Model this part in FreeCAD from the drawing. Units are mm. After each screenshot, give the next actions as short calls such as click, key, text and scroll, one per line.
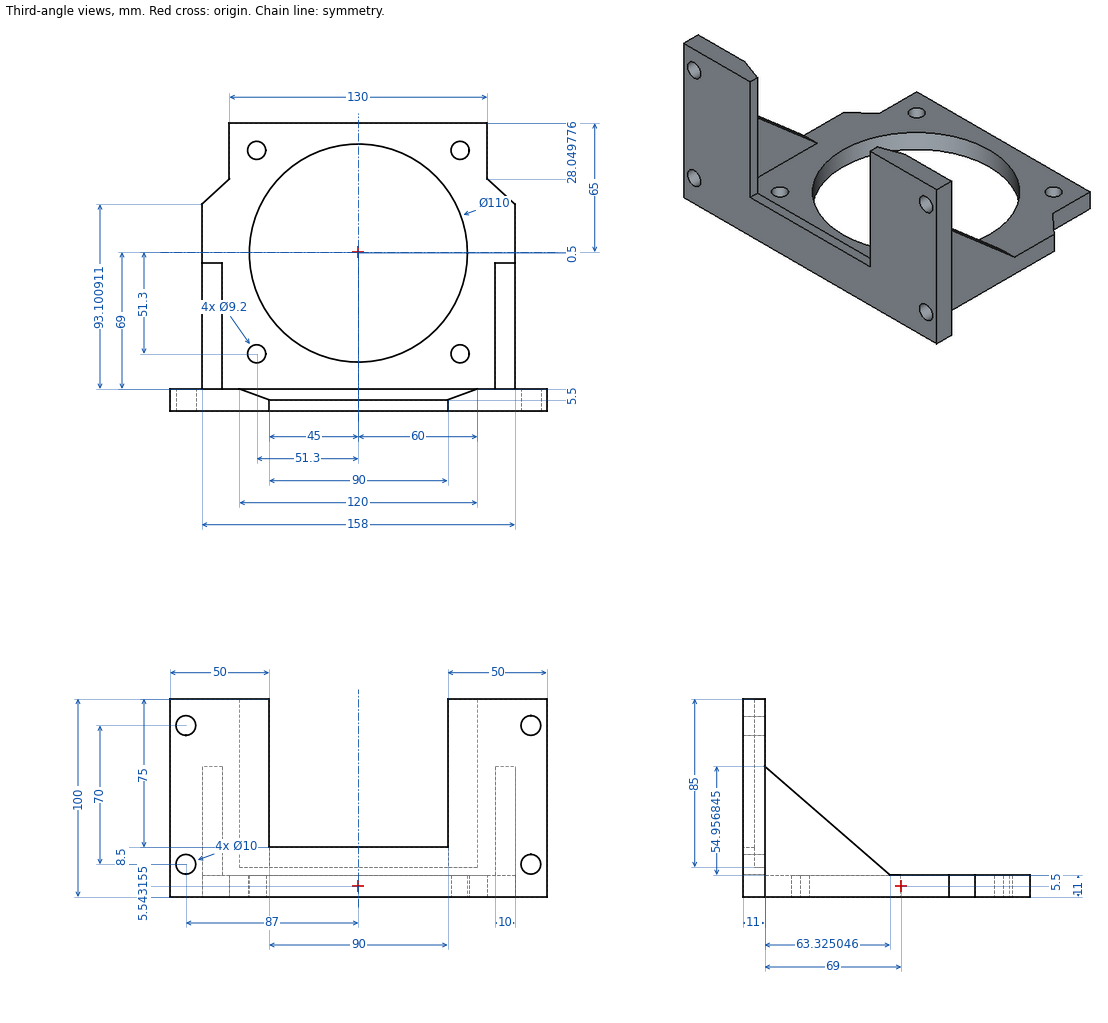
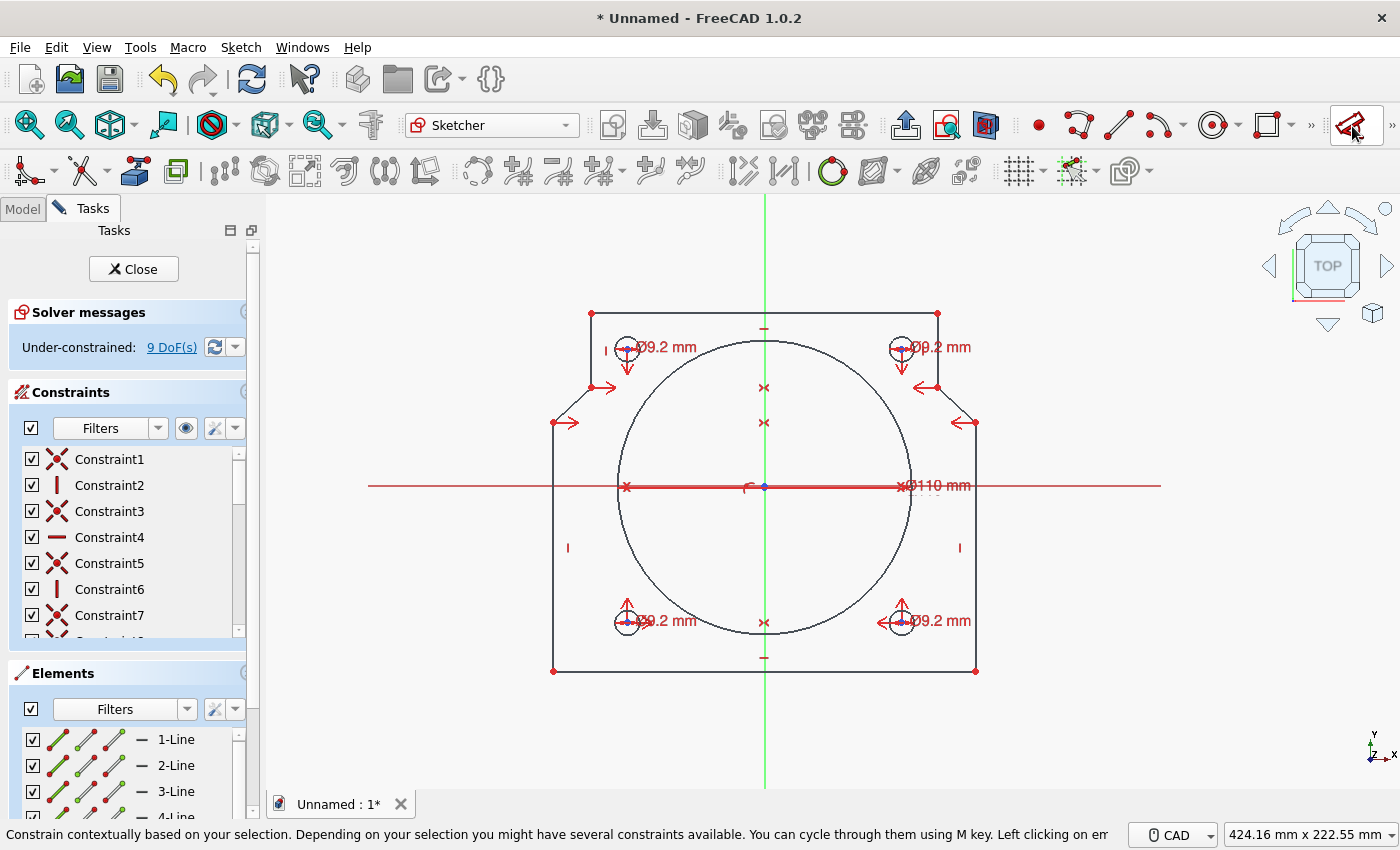
click(680, 672)
click(667, 706)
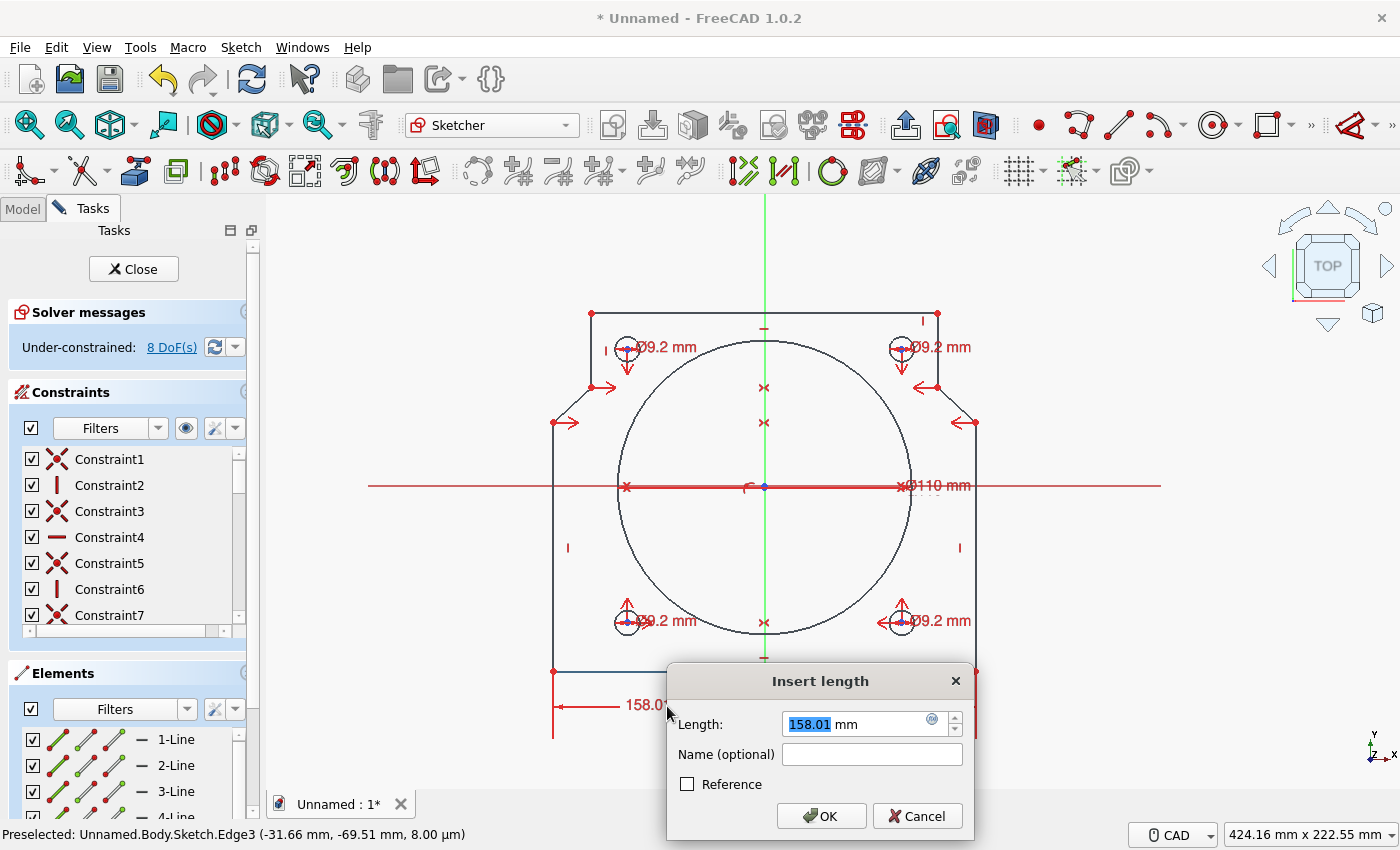
text(158)
key(Return)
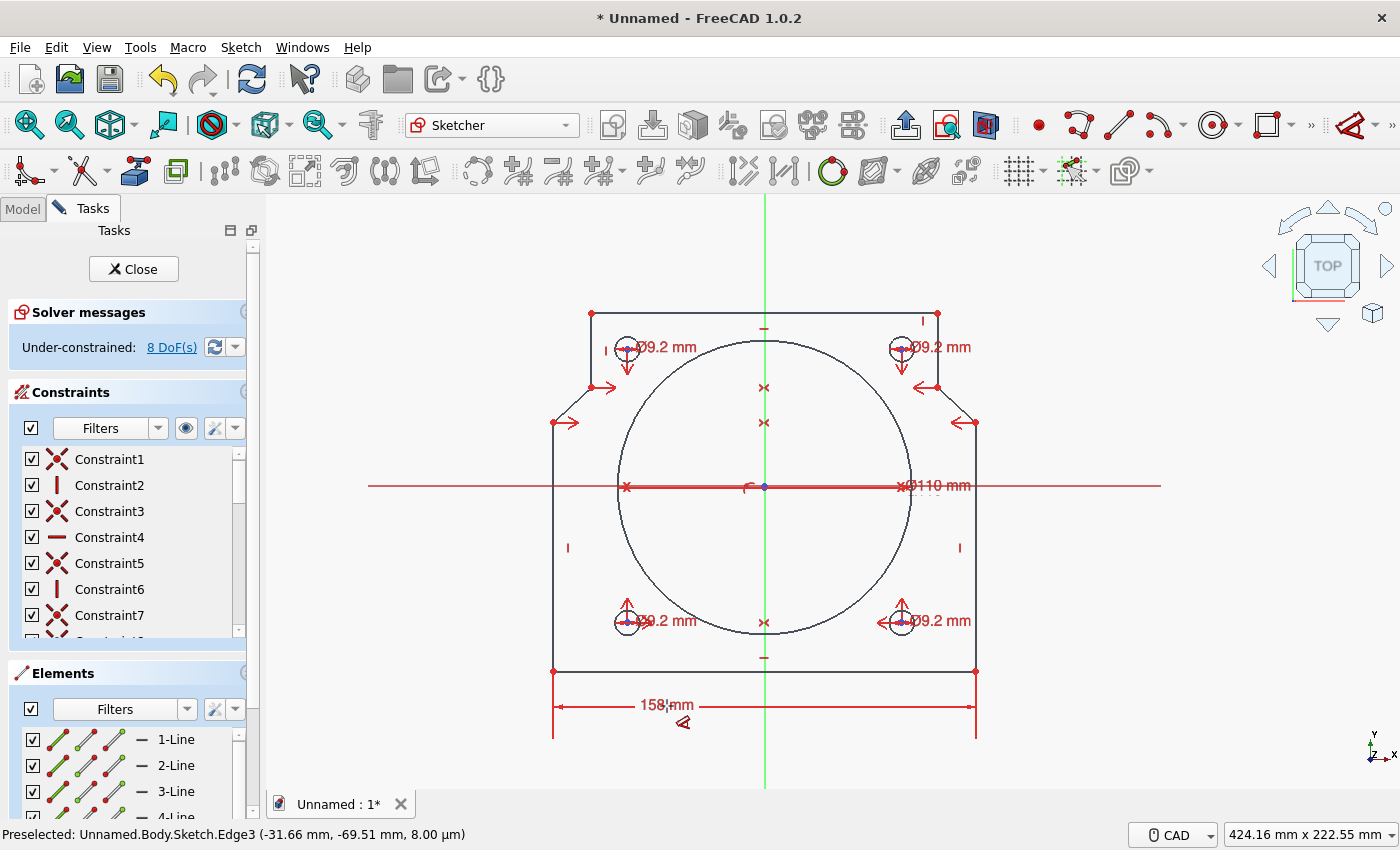
click(834, 313)
click(685, 279)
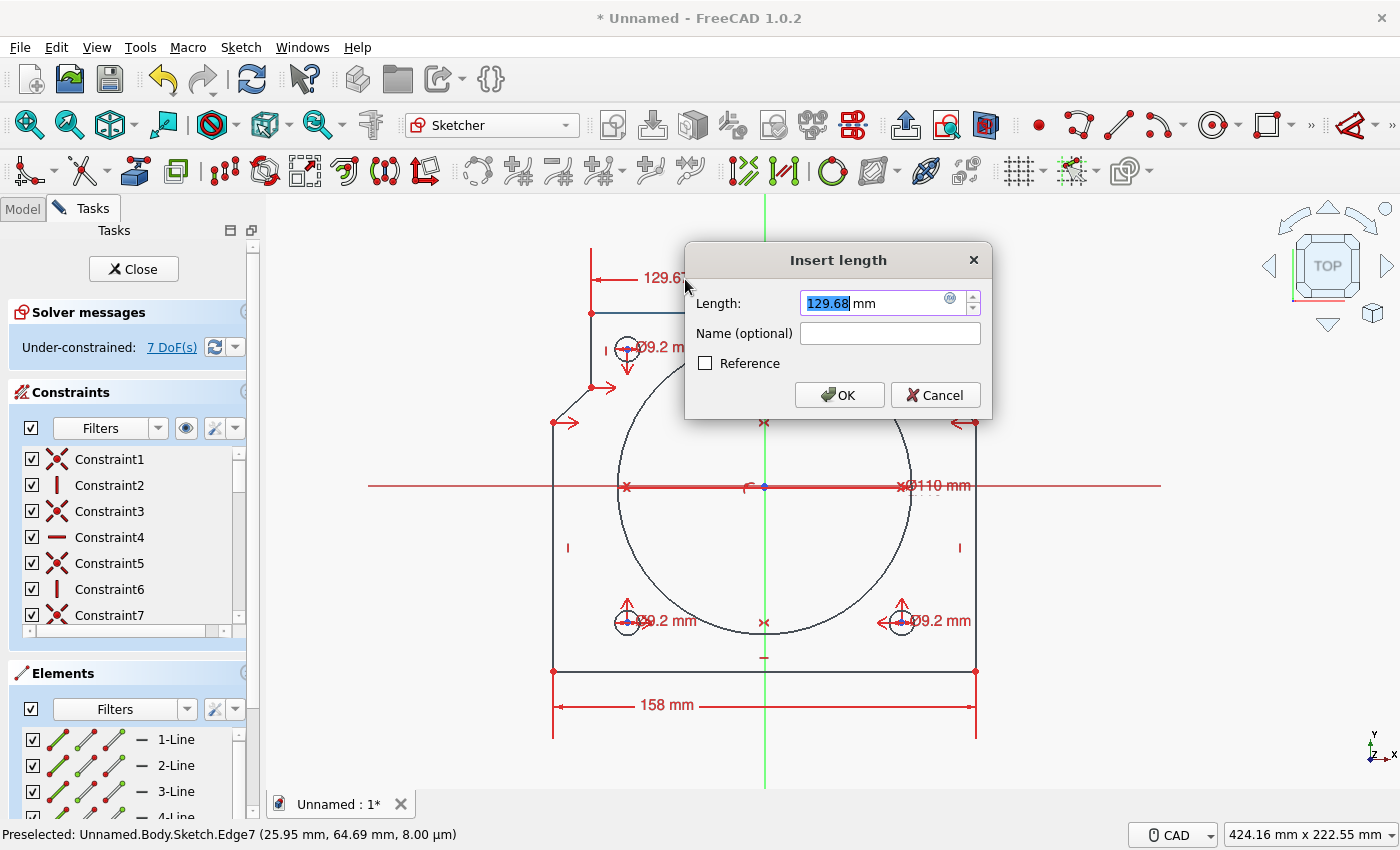
text(130)
key(Return)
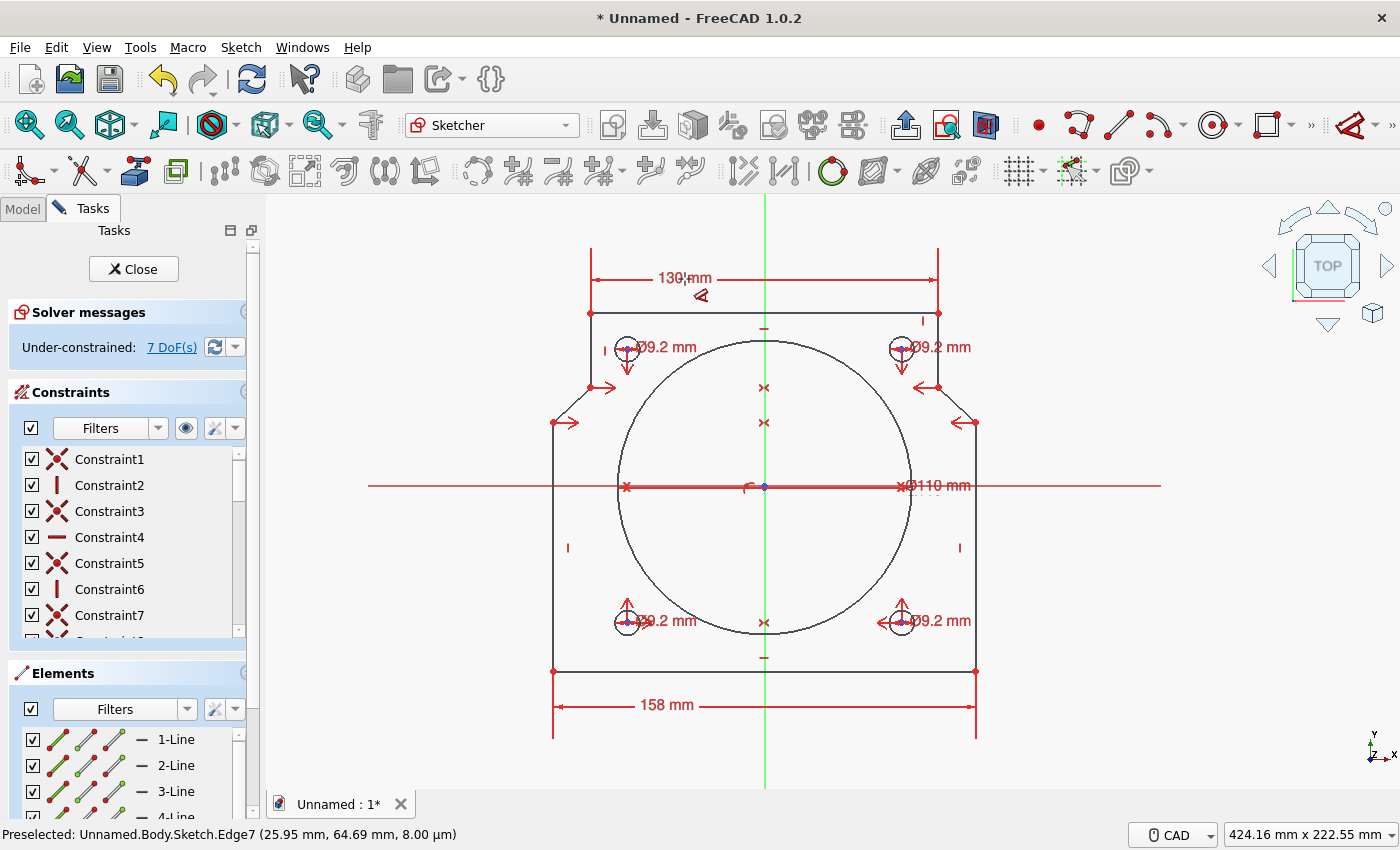
click(553, 672)
click(519, 579)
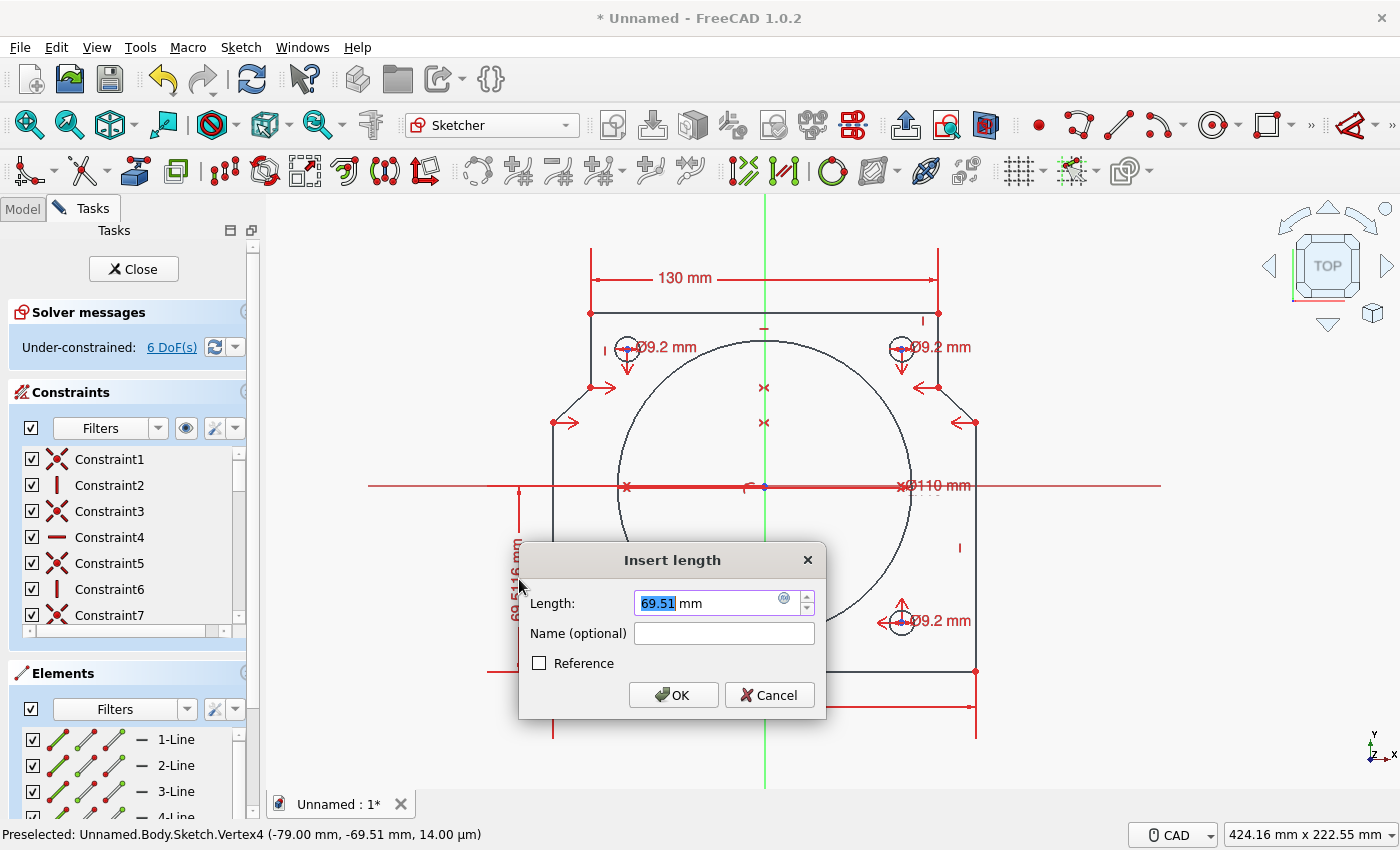
text(69)
key(Return)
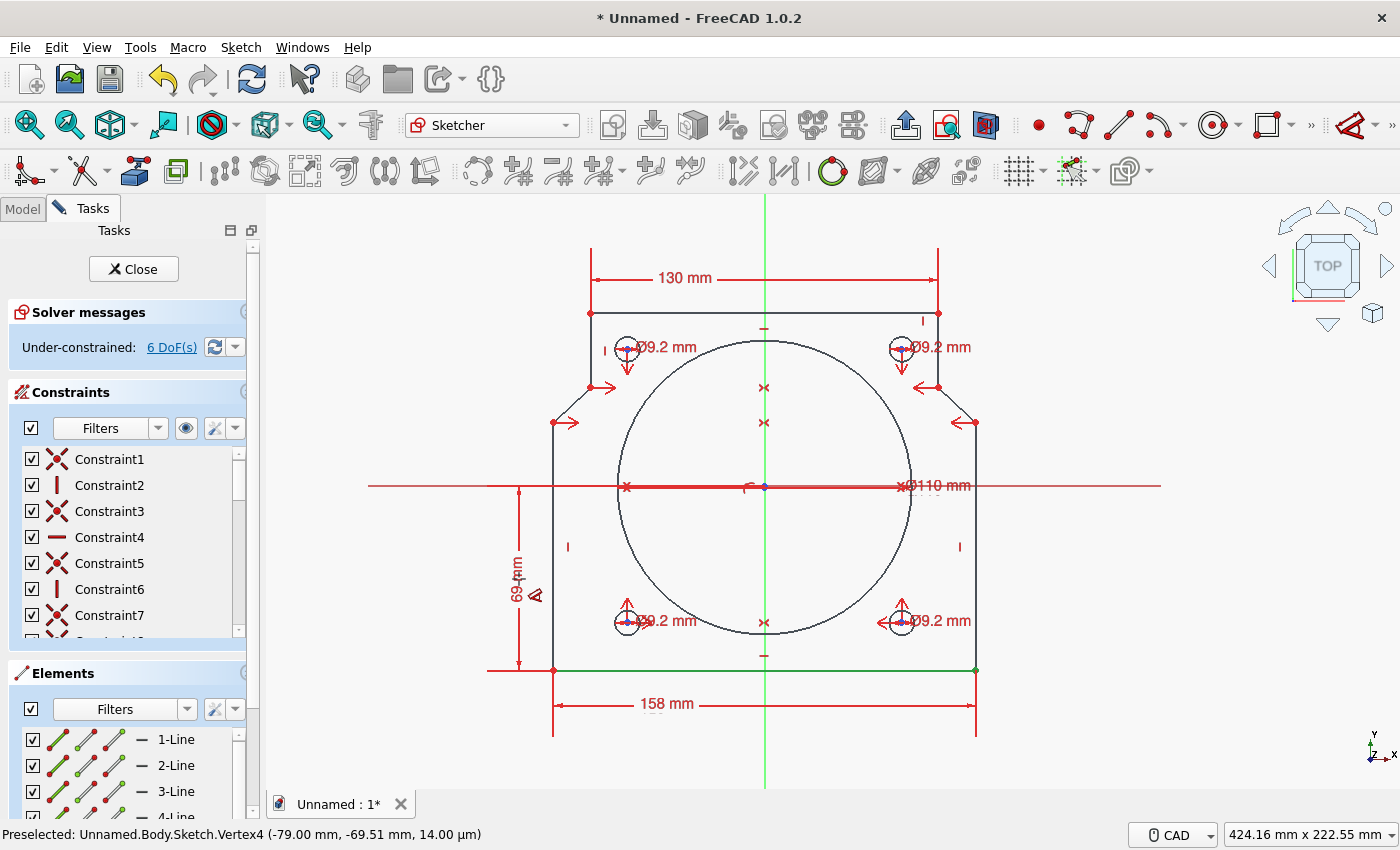
click(938, 313)
click(972, 400)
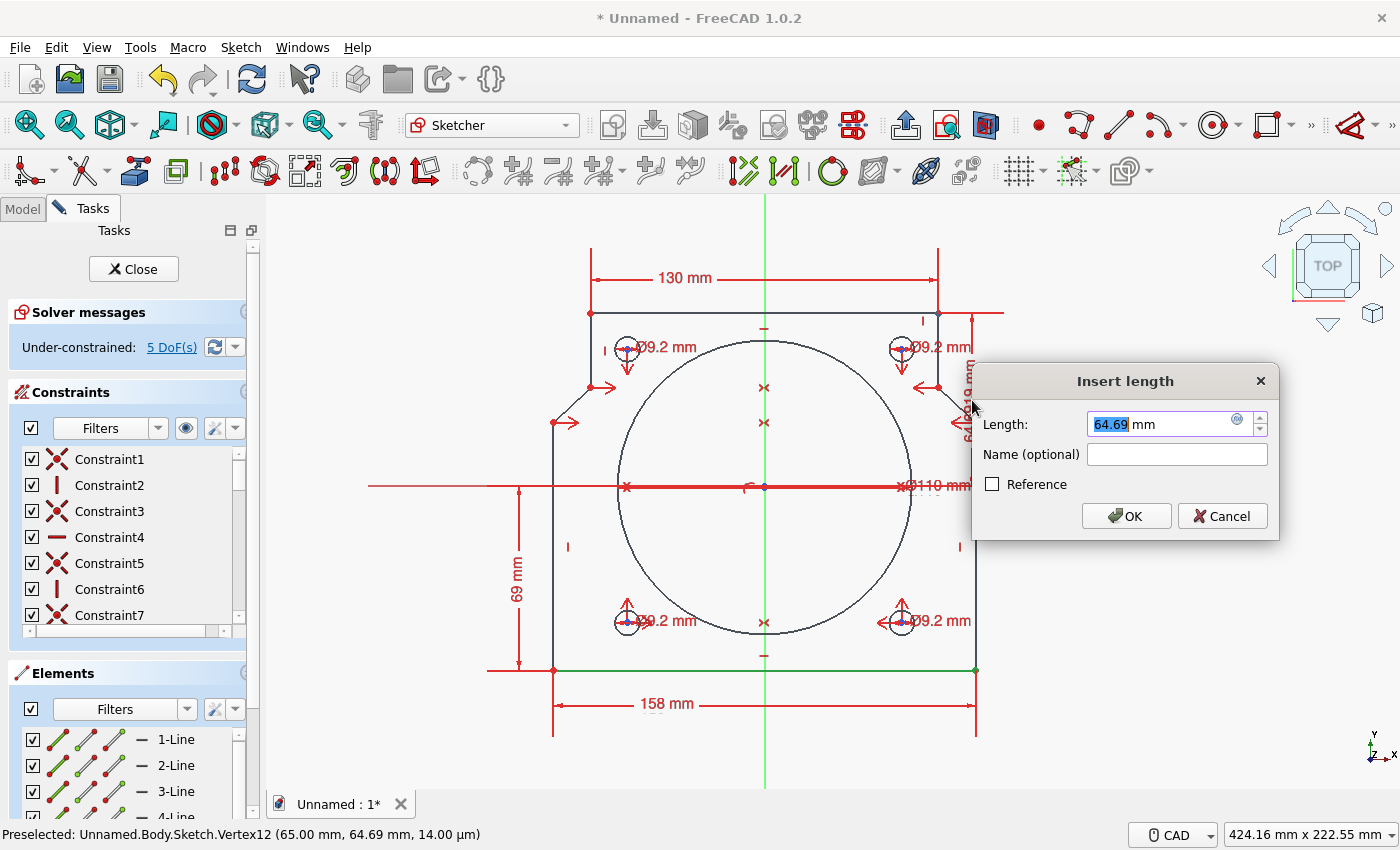
text(65)
key(Return)